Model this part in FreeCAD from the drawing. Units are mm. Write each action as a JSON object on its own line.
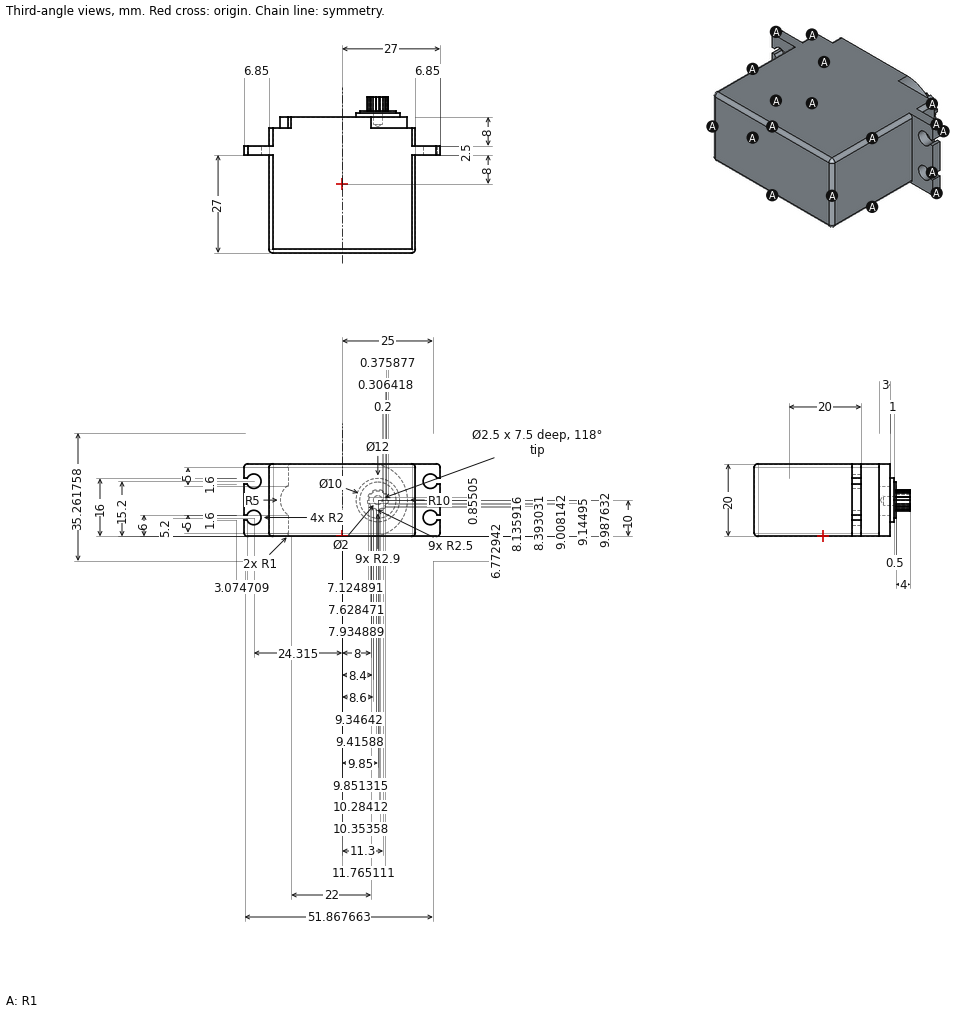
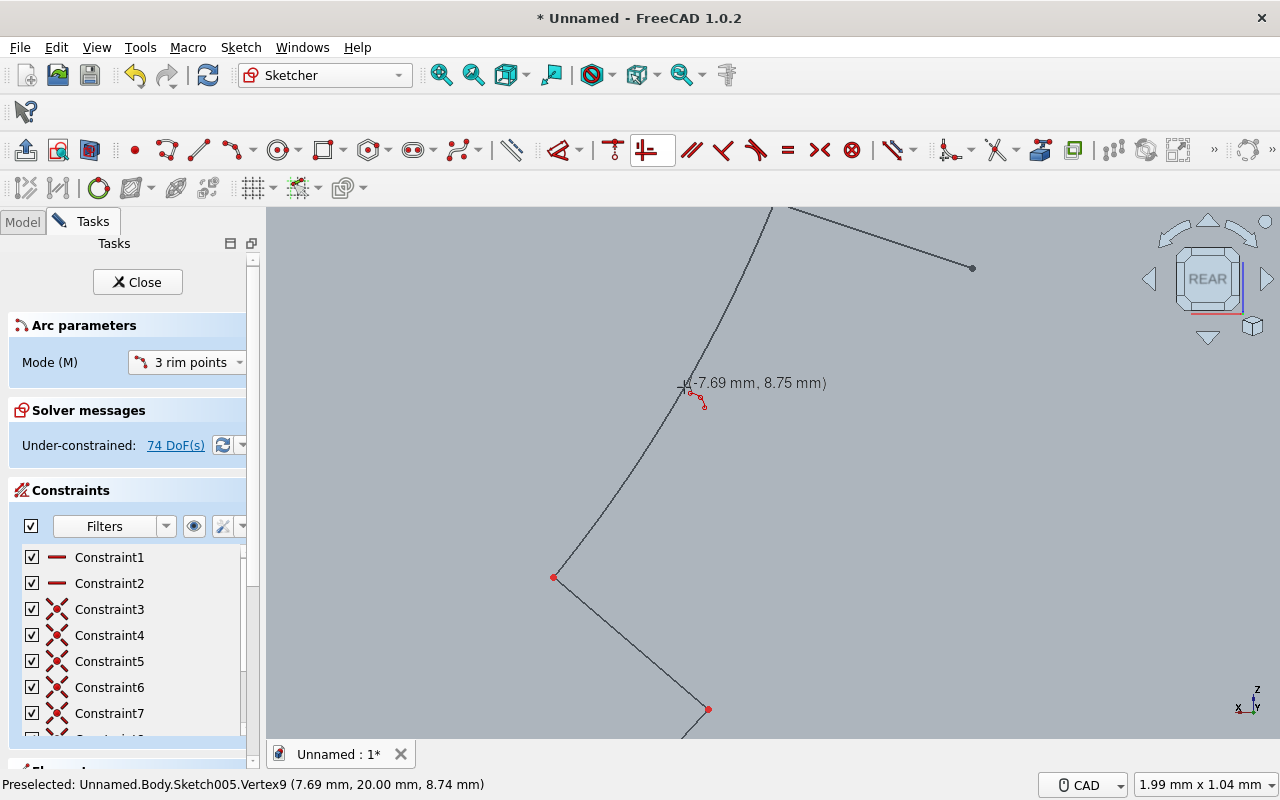
{"action": "scroll", "coordinate": [671, 415], "scroll_direction": "down", "scroll_amount": 15}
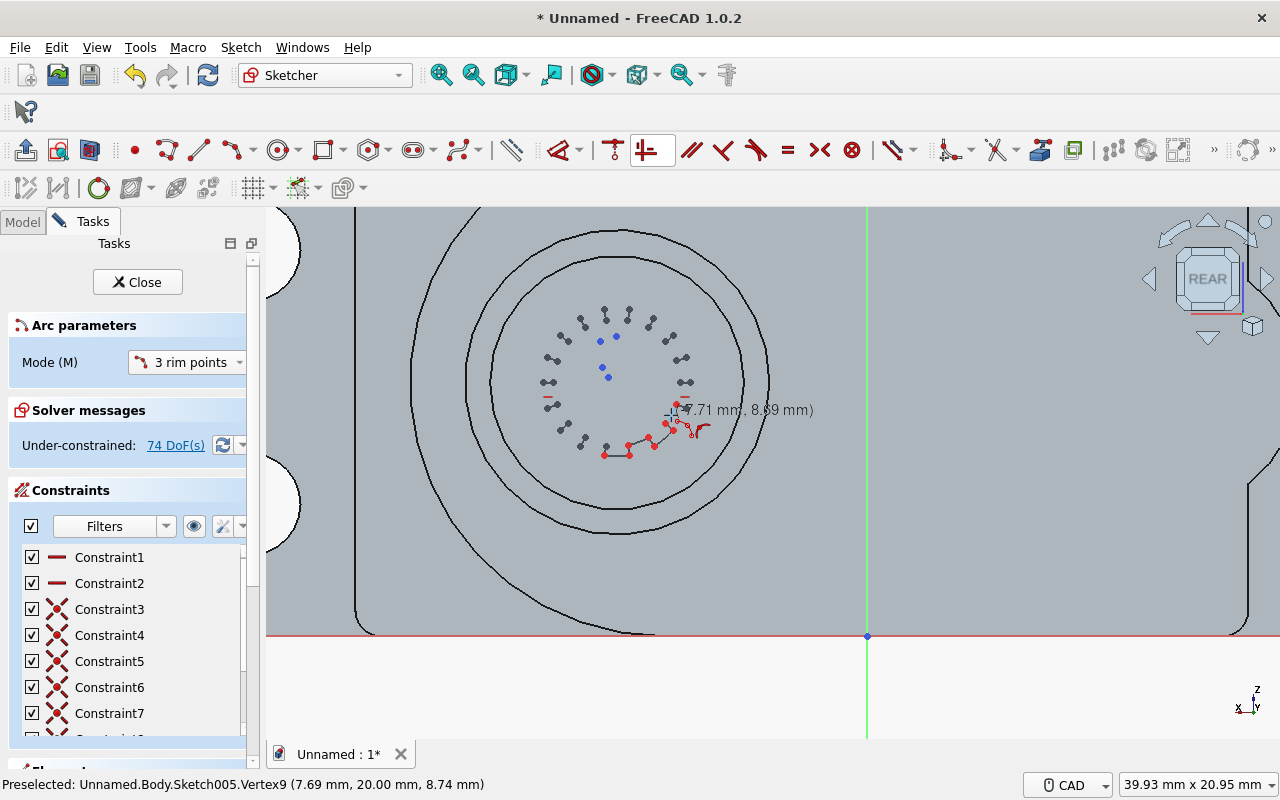
{"action": "scroll", "coordinate": [686, 407], "scroll_direction": "up", "scroll_amount": 6}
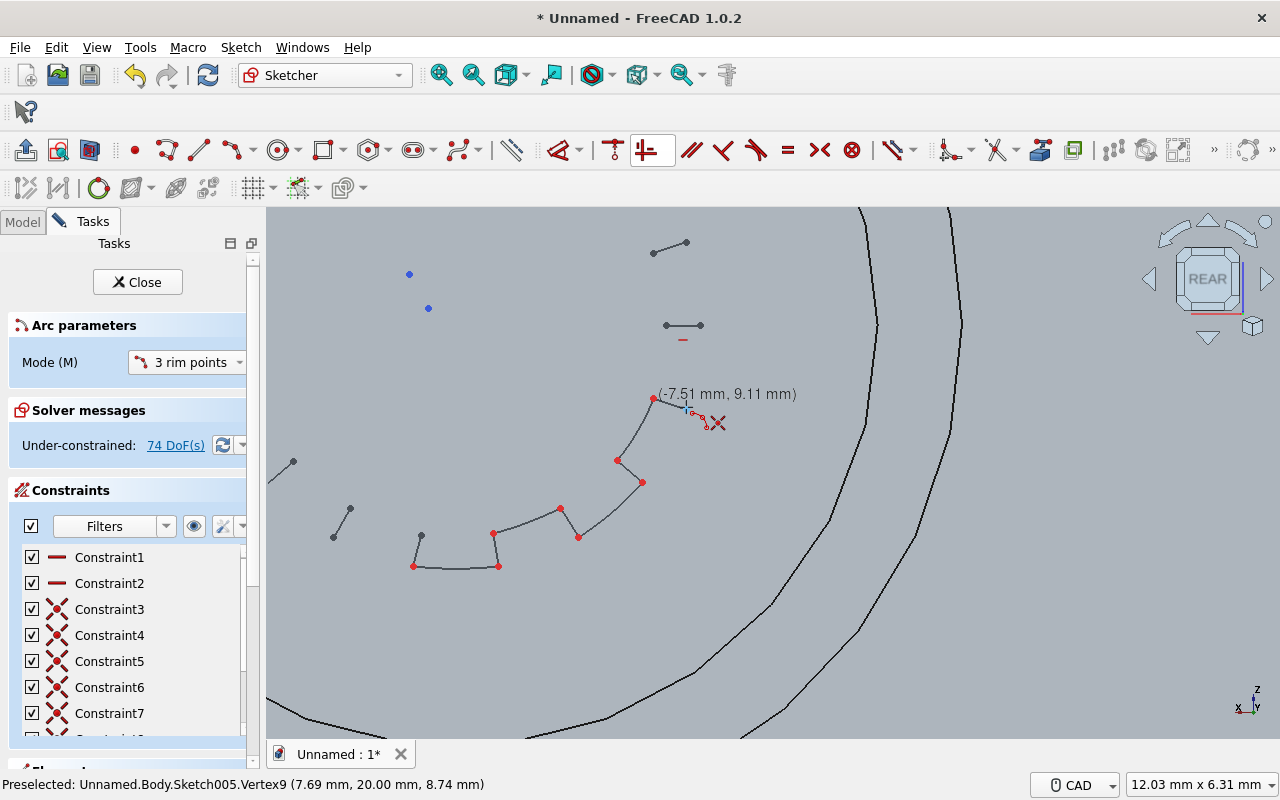
{"action": "left_click", "coordinate": [686, 410]}
{"action": "left_click", "coordinate": [701, 326]}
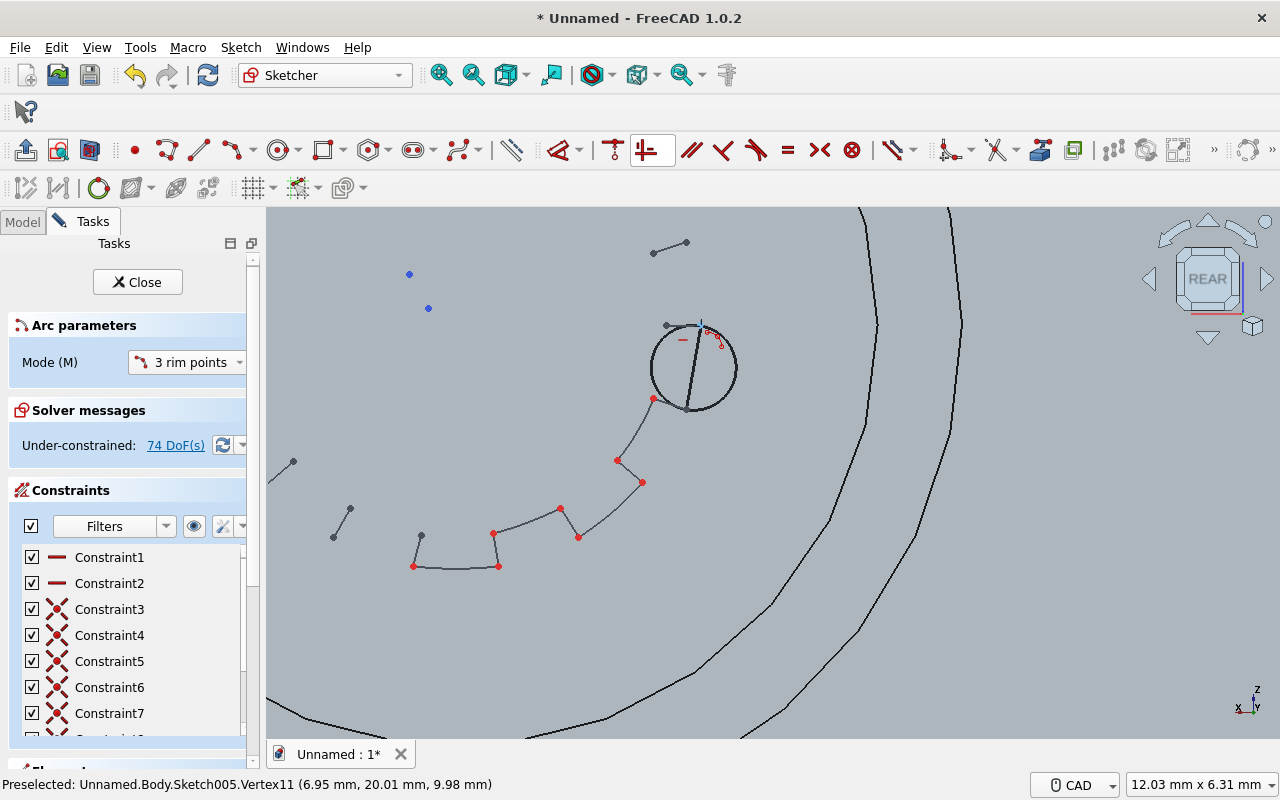
{"action": "scroll", "coordinate": [697, 366], "scroll_direction": "up", "scroll_amount": 8}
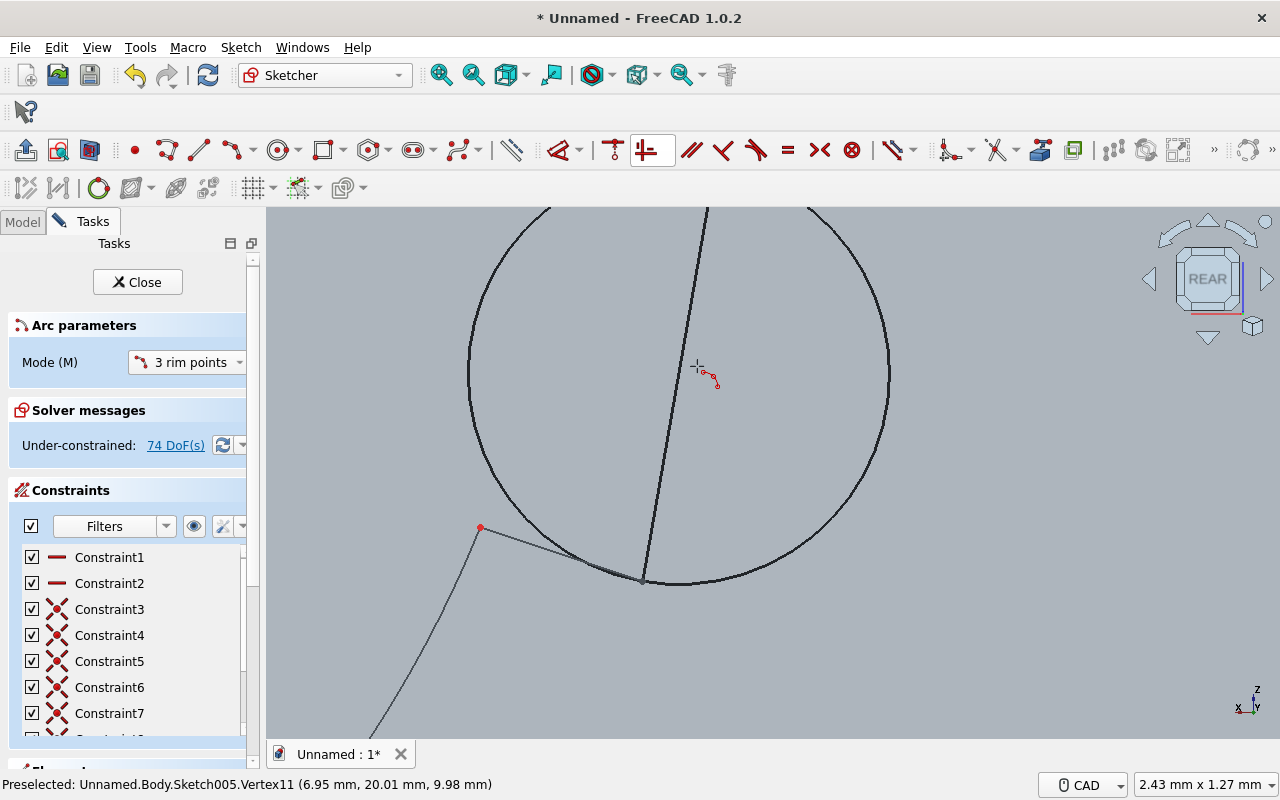
{"action": "left_click", "coordinate": [695, 367]}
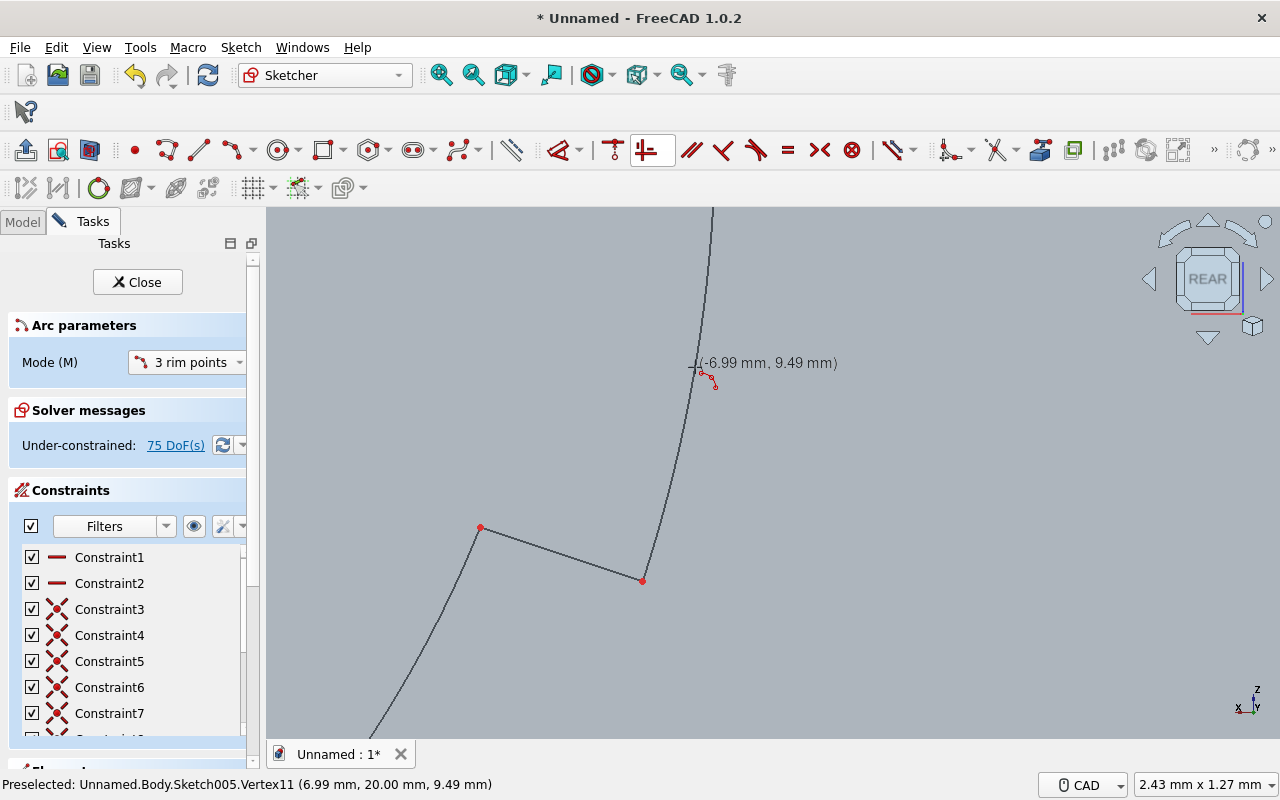
{"action": "scroll", "coordinate": [688, 397], "scroll_direction": "down", "scroll_amount": 14}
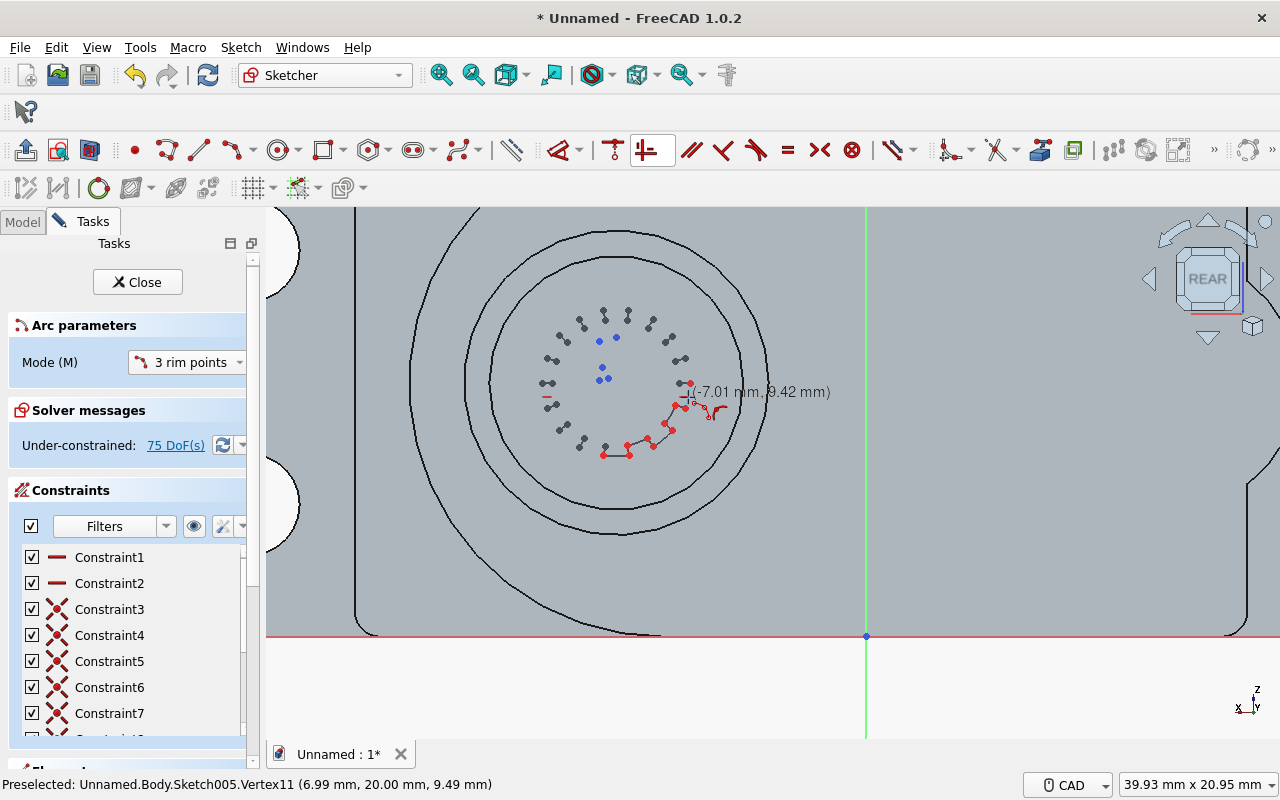
{"action": "scroll", "coordinate": [680, 383], "scroll_direction": "up", "scroll_amount": 6}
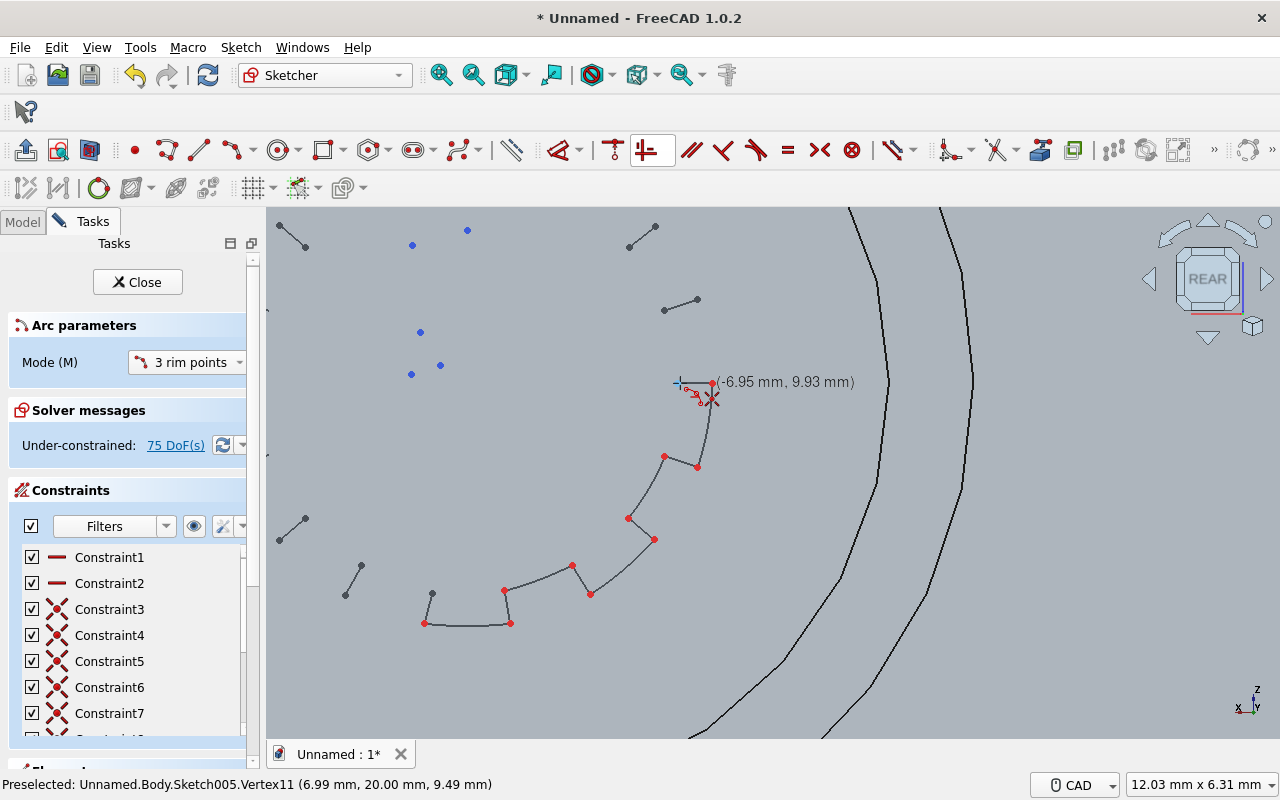
{"action": "left_click", "coordinate": [678, 383]}
{"action": "left_click", "coordinate": [665, 310]}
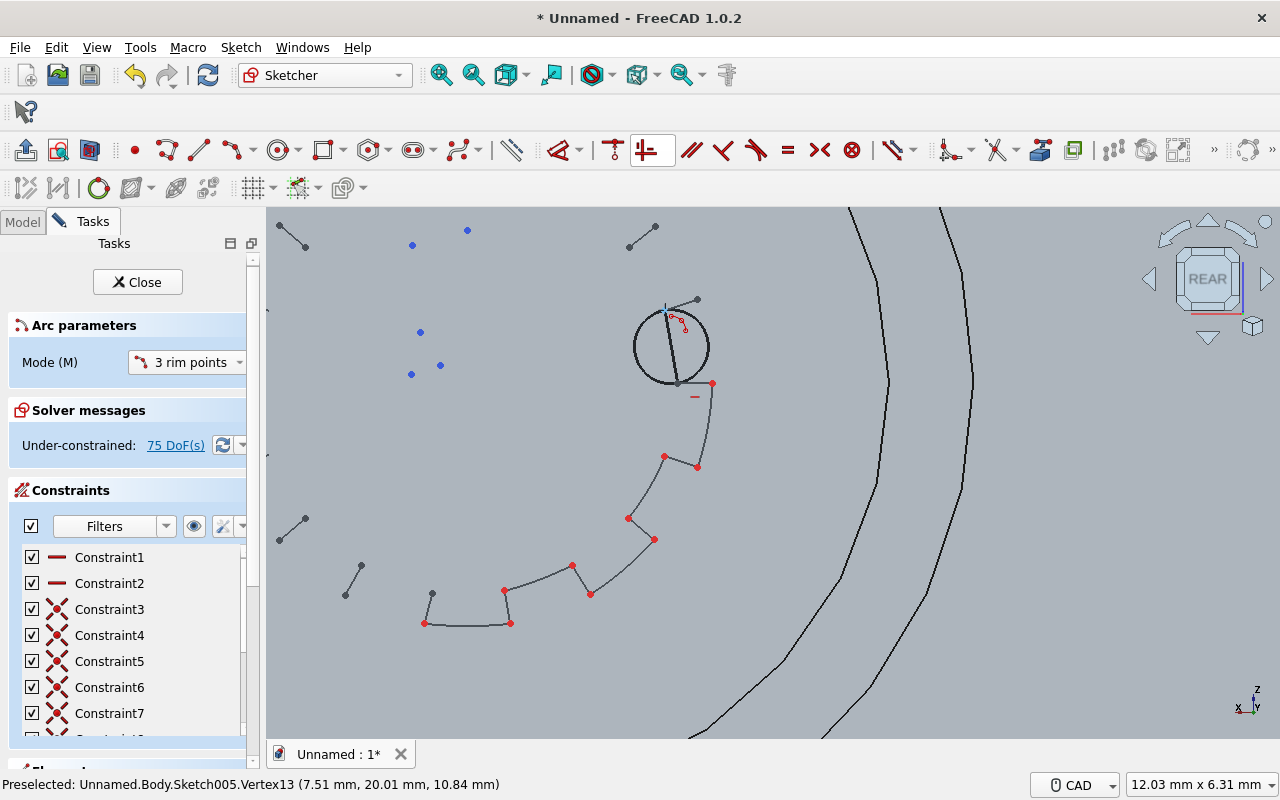
{"action": "scroll", "coordinate": [675, 345], "scroll_direction": "up", "scroll_amount": 9}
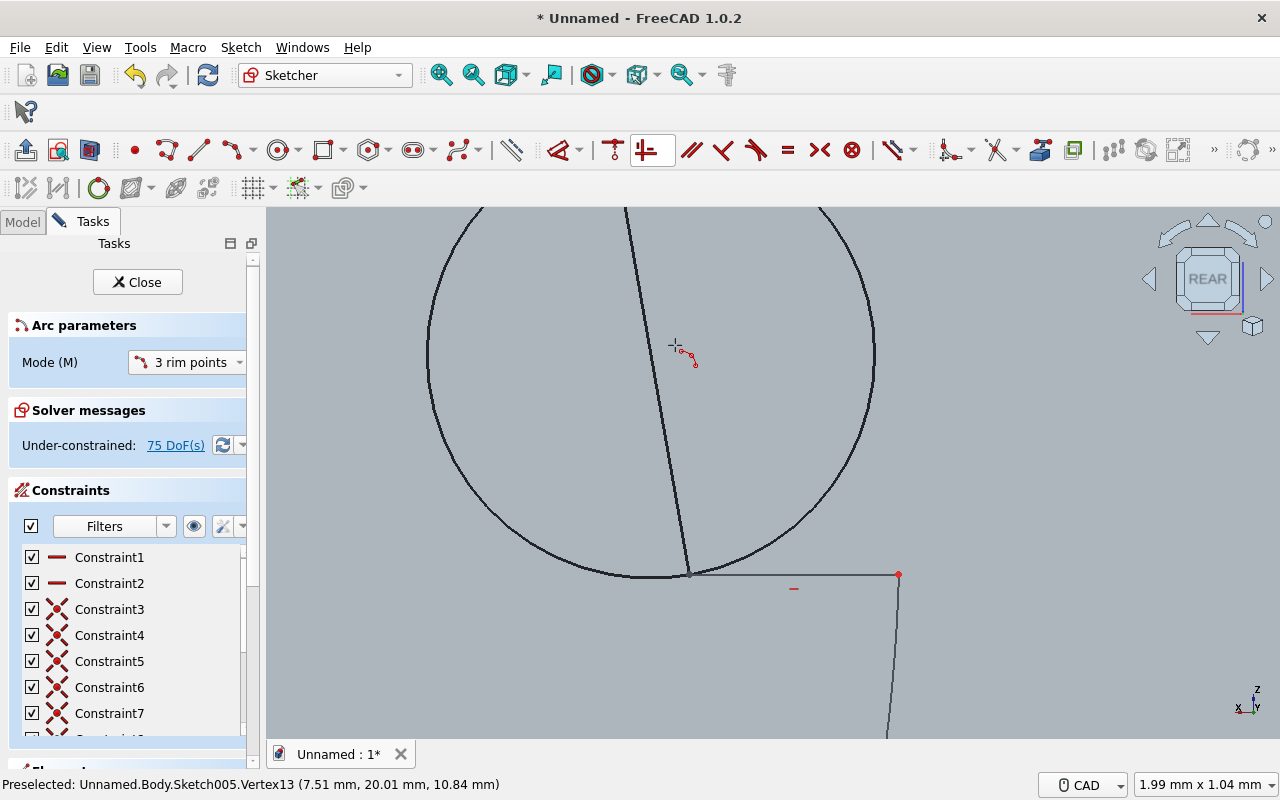
{"action": "left_click", "coordinate": [674, 342]}